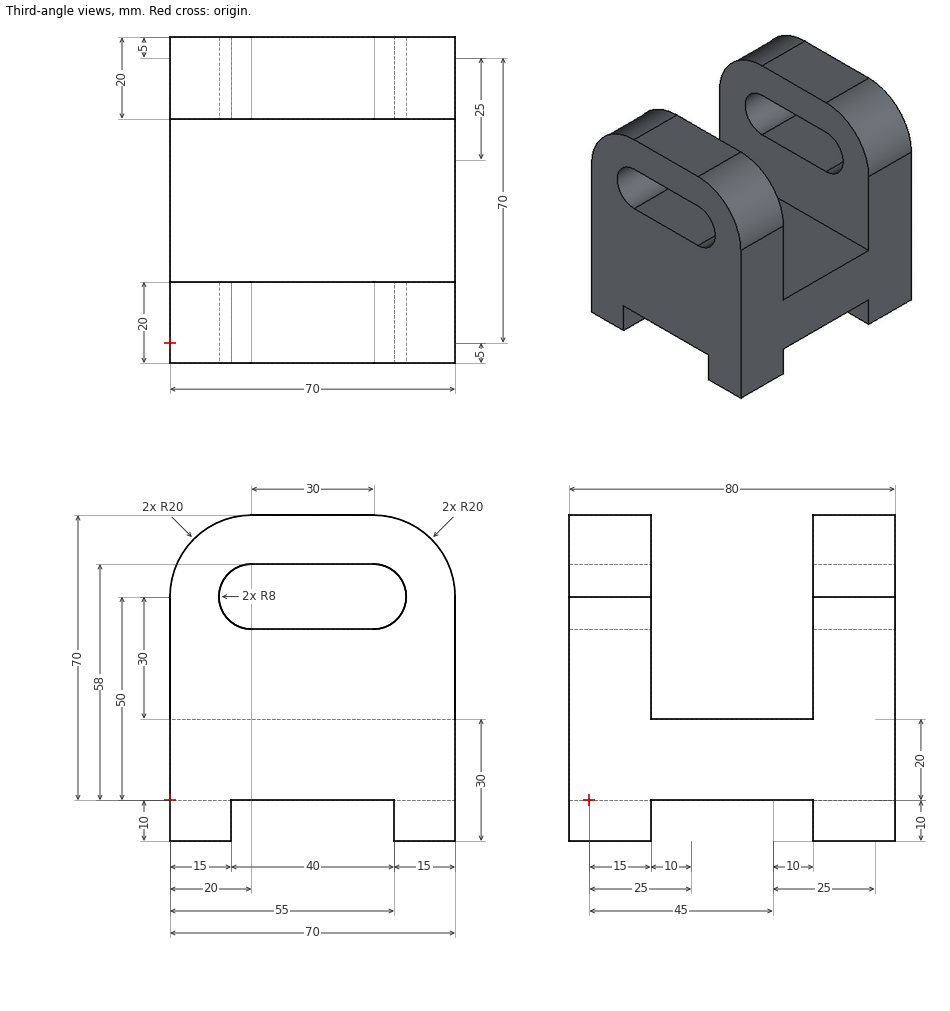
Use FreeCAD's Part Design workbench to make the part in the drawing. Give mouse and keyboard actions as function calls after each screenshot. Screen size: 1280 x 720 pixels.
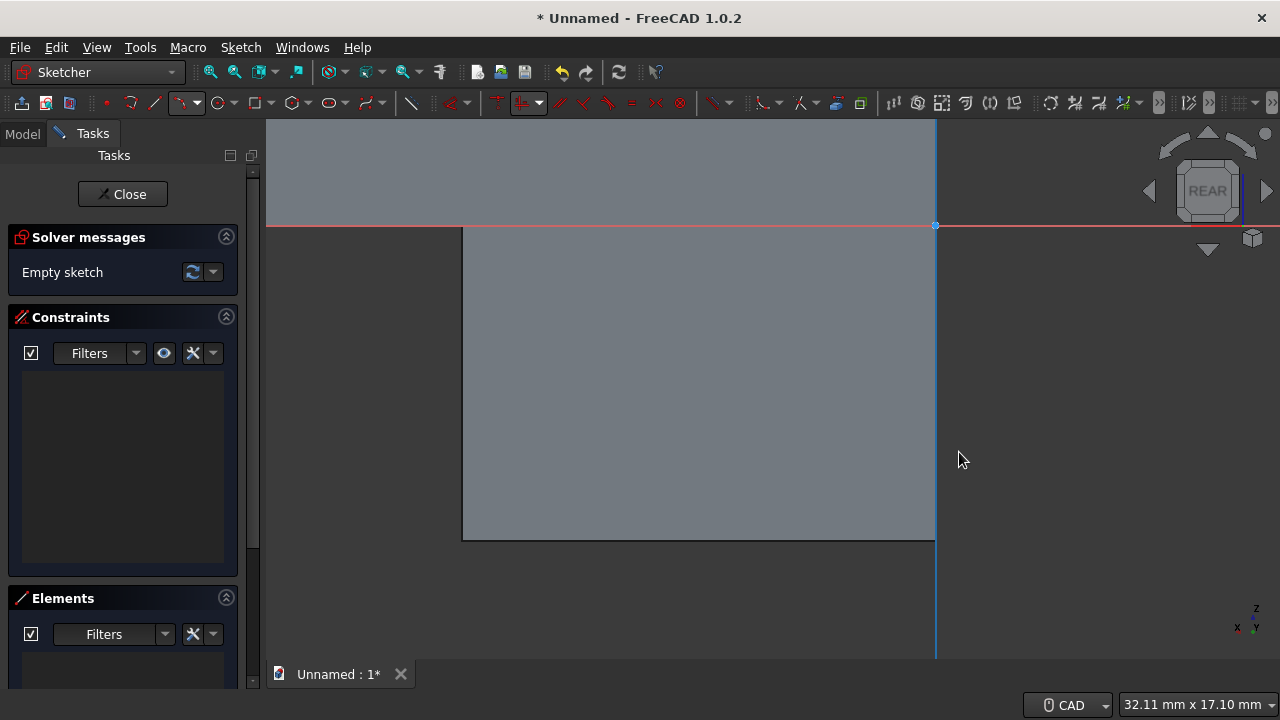
key(g)
key(r)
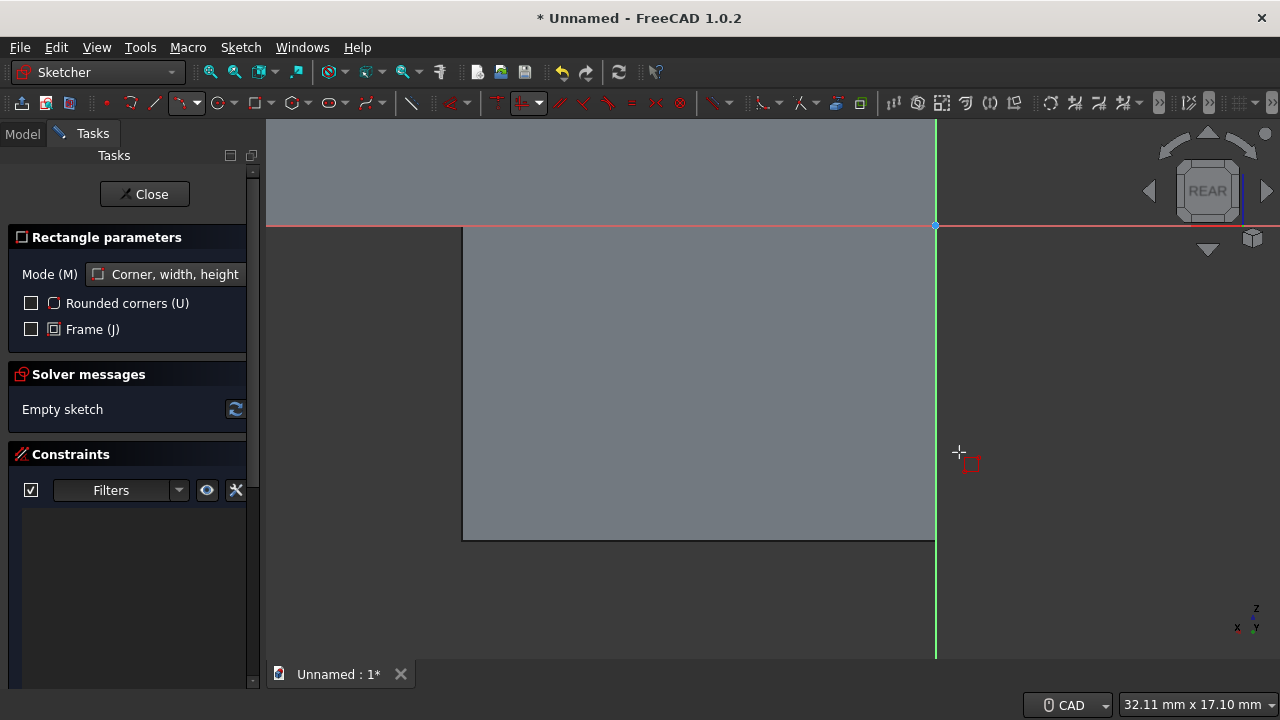
click(936, 226)
click(462, 541)
key(Escape)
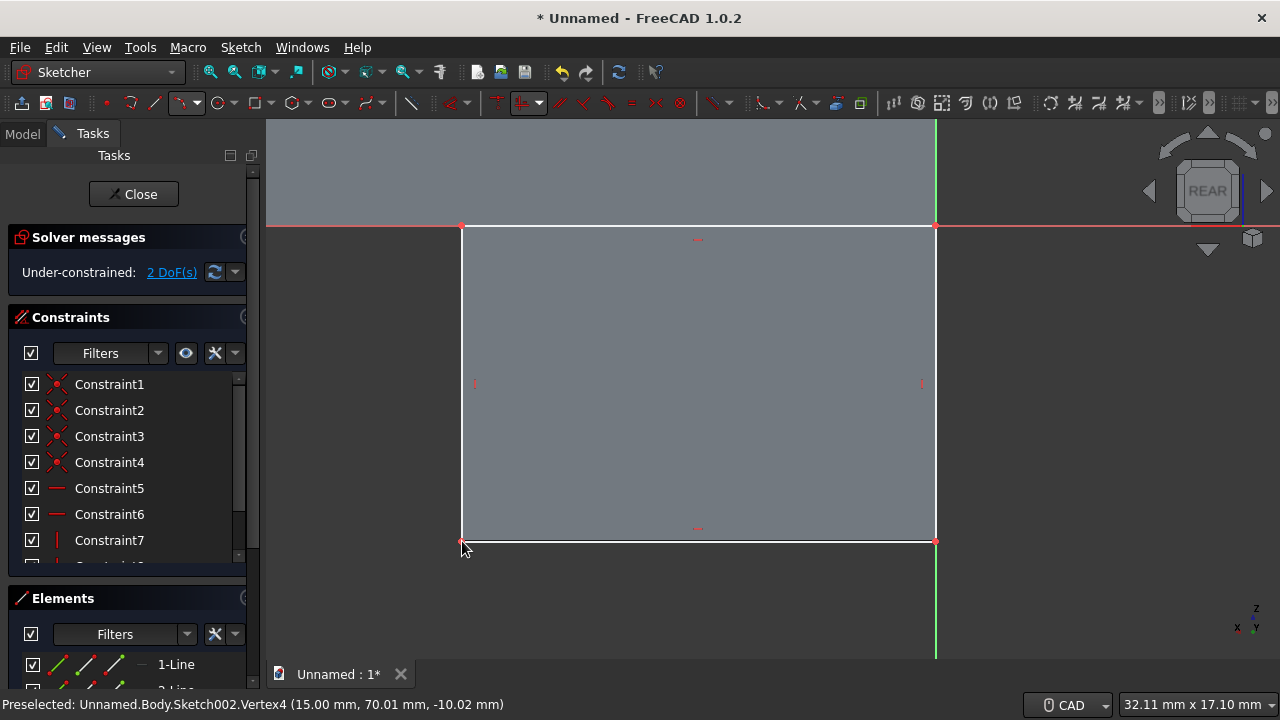
key(d)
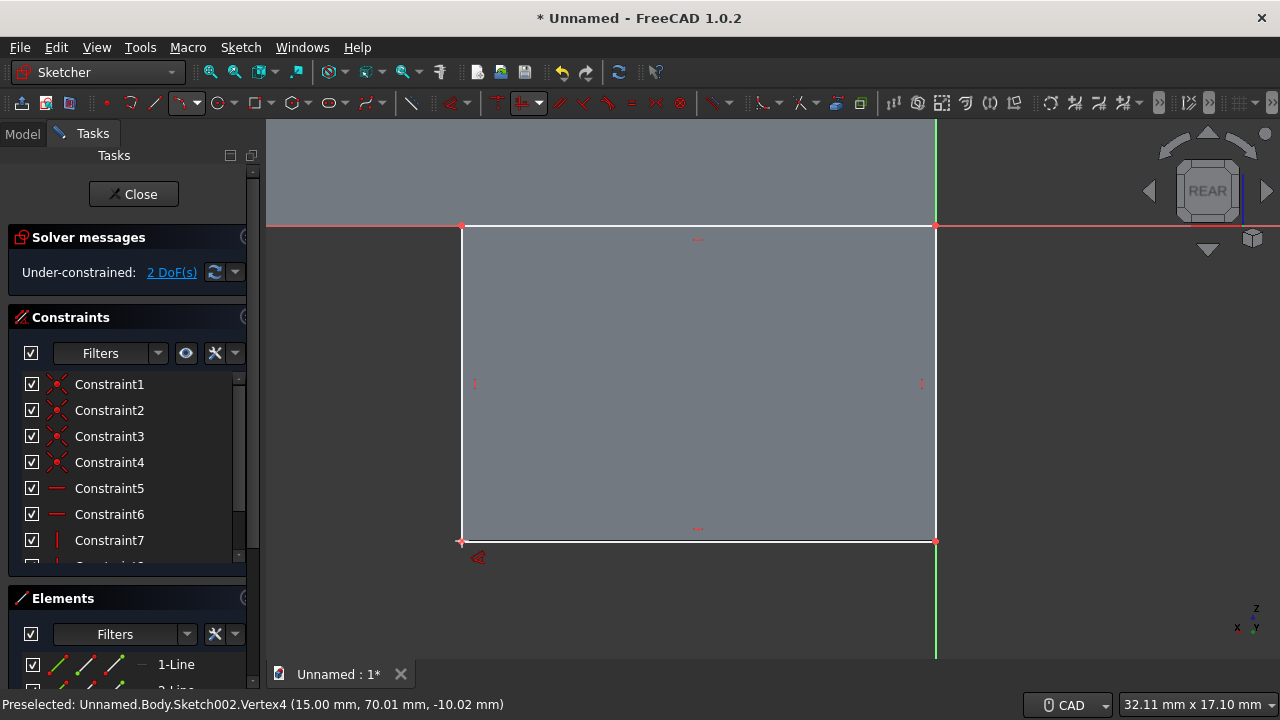
click(794, 226)
click(699, 192)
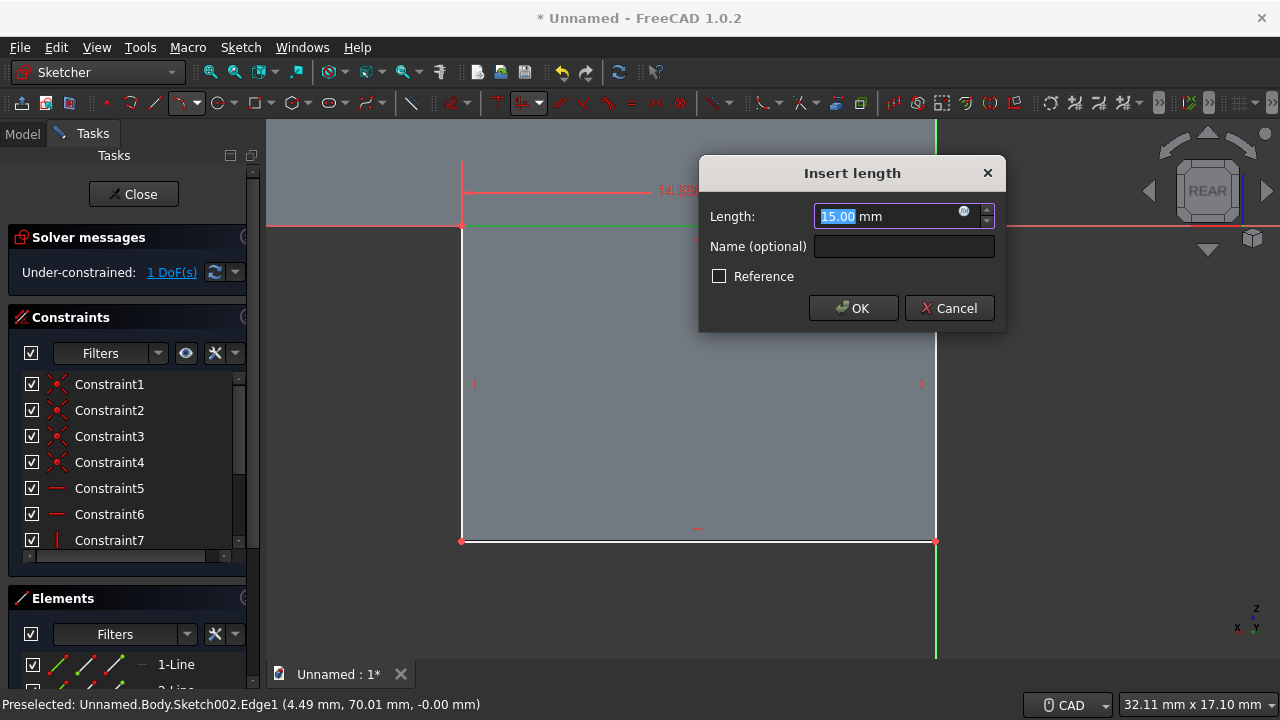
text(15)
key(Return)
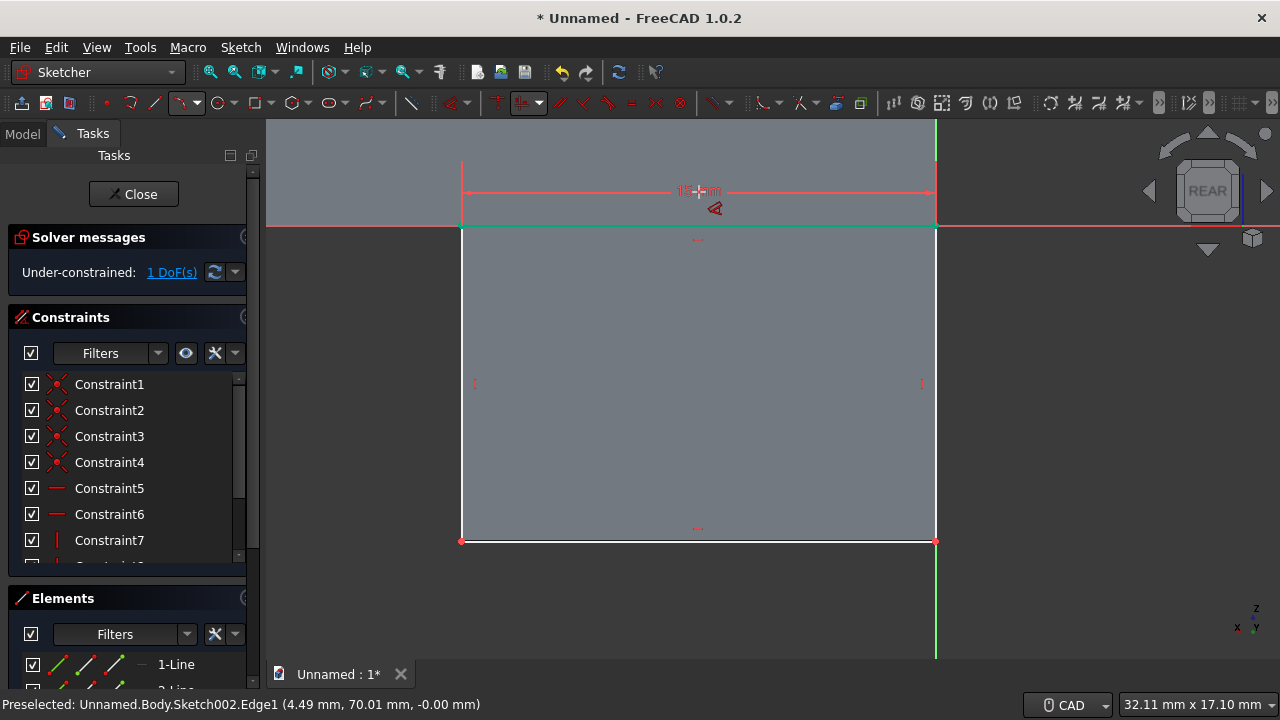
click(462, 321)
click(428, 384)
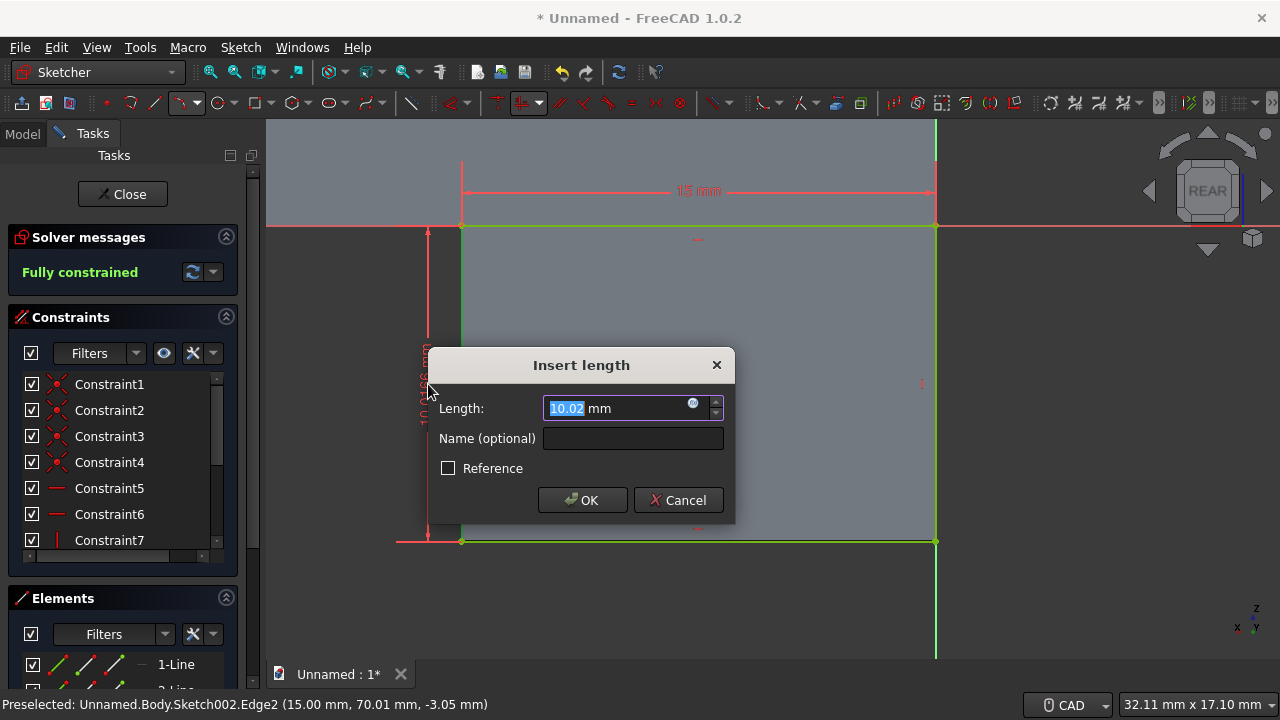
text(10)
key(Return)
key(Escape)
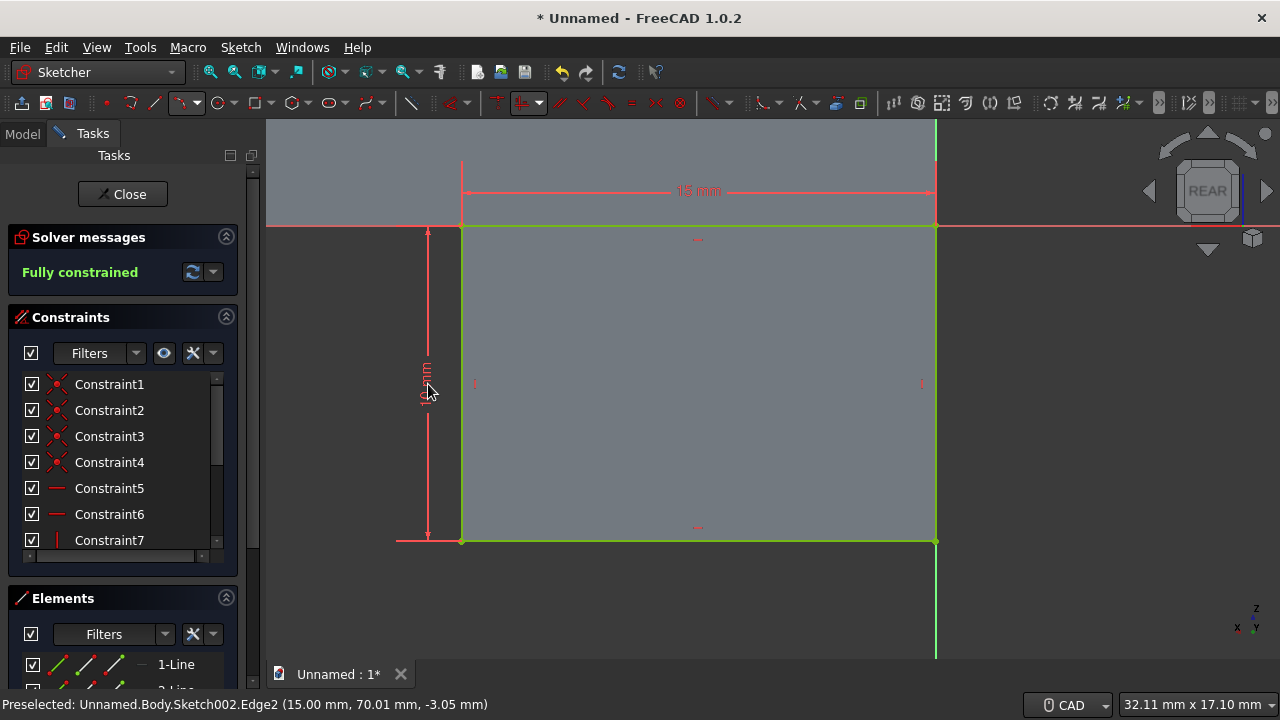
click(123, 194)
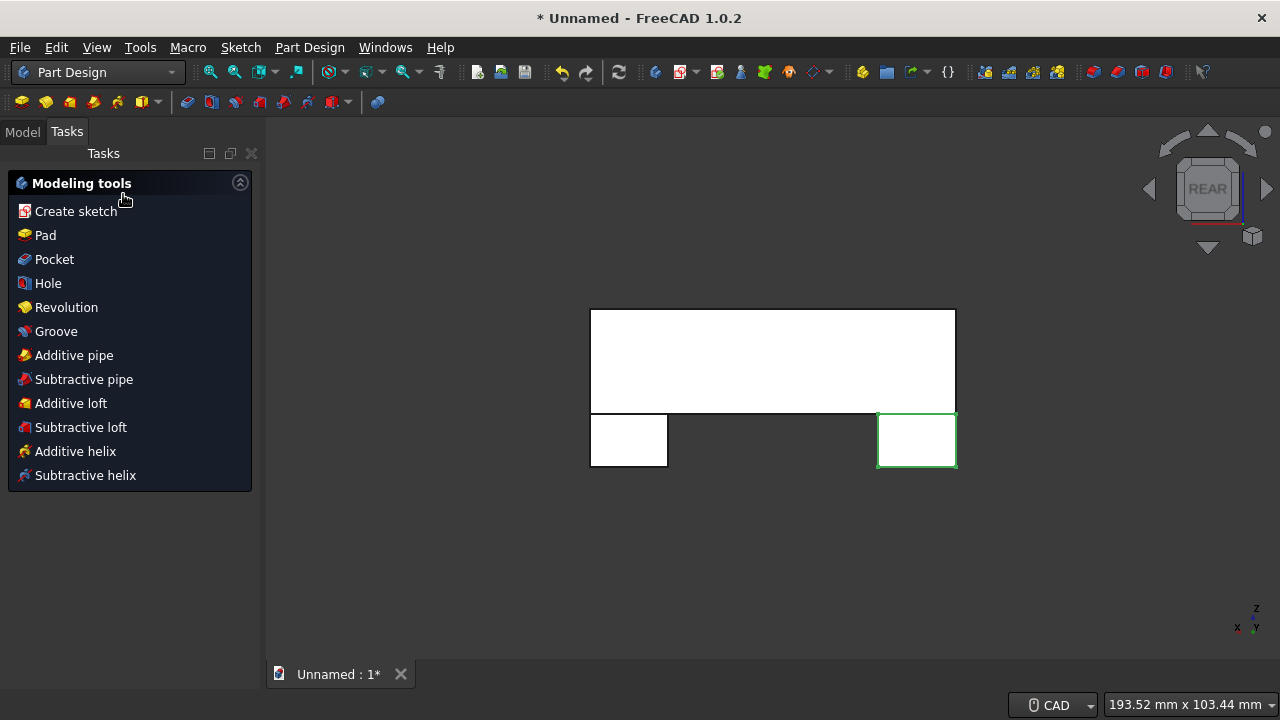
click(22, 102)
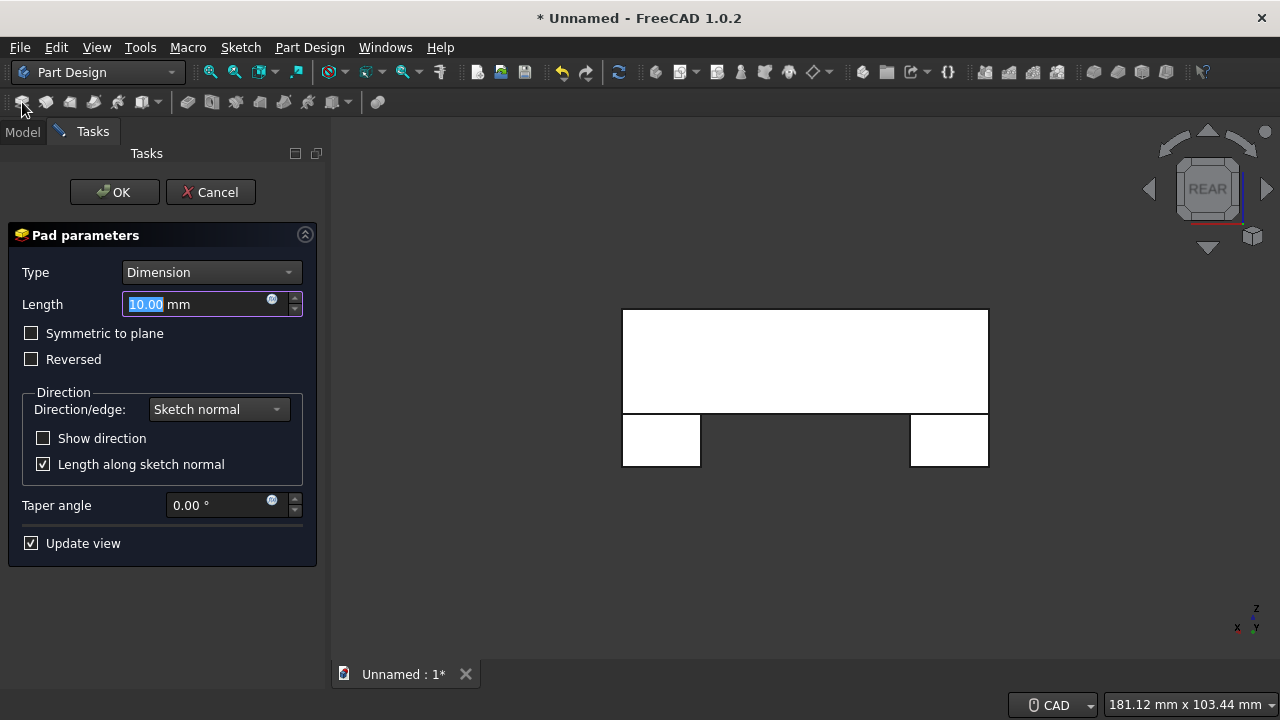
text(25)
key(Tab)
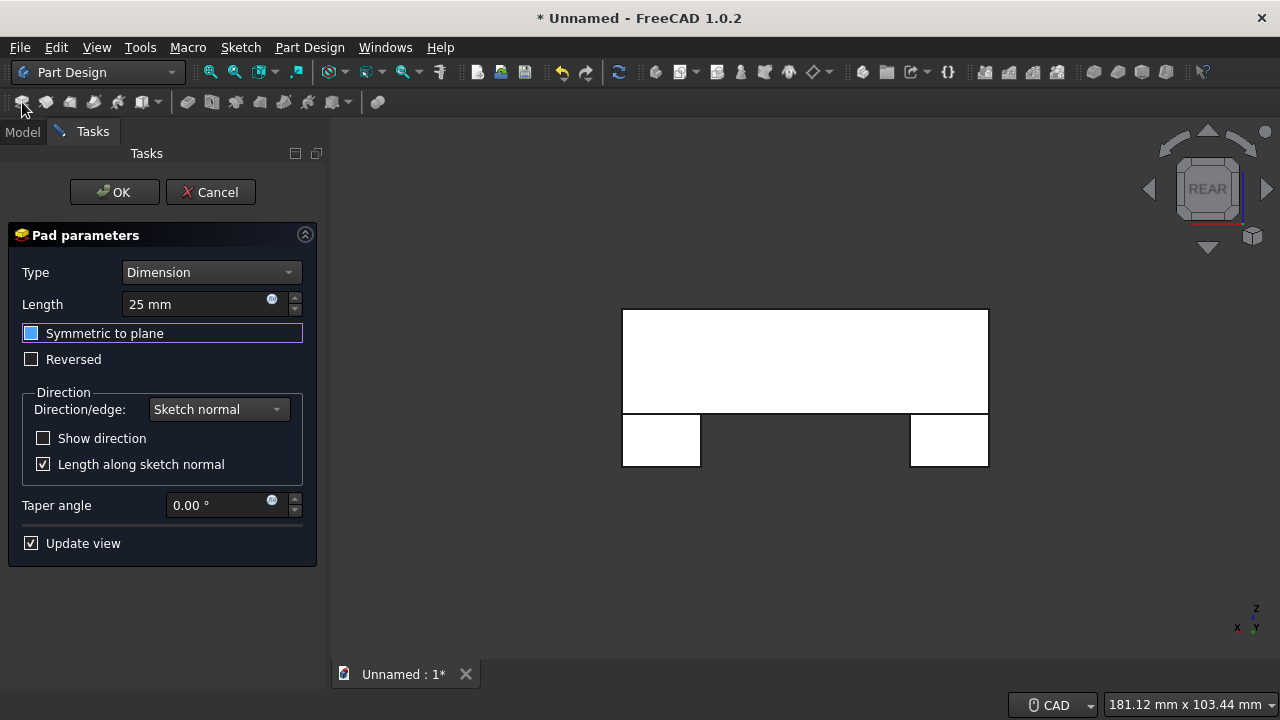
click(30, 359)